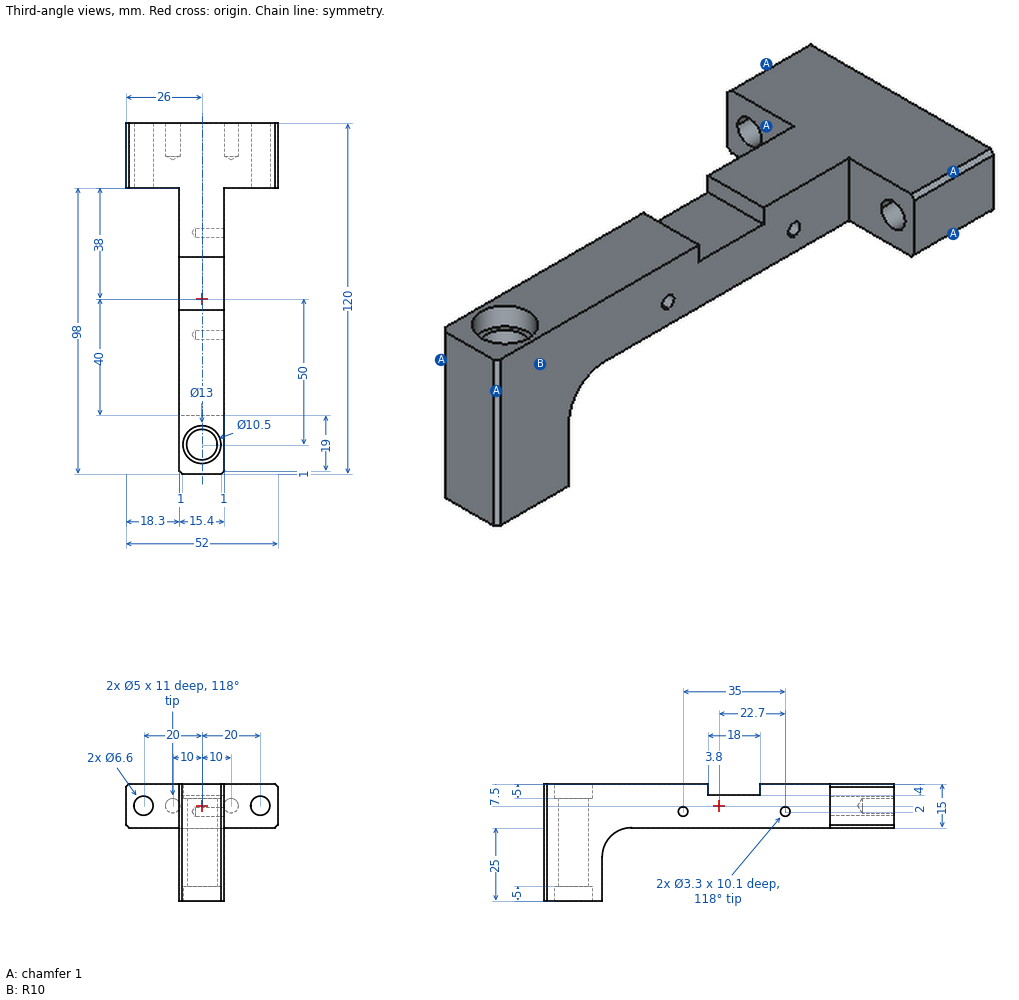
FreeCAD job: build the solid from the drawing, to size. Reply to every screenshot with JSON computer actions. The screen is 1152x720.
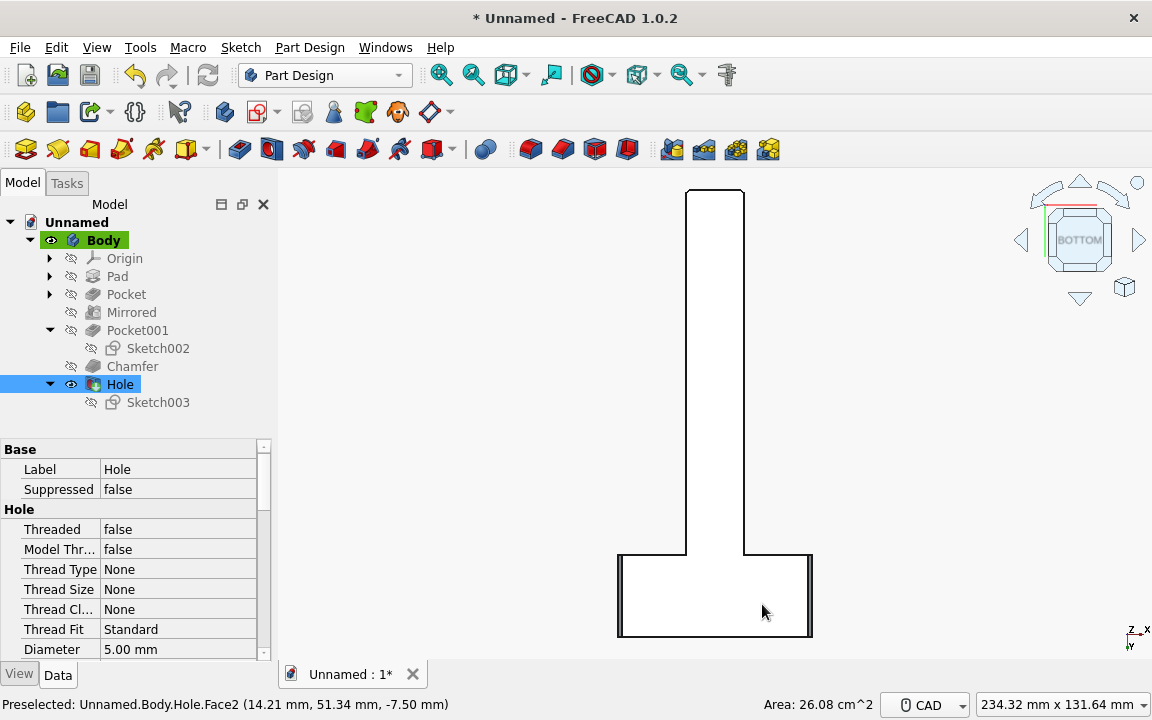
{"action": "left_click", "coordinate": [258, 112]}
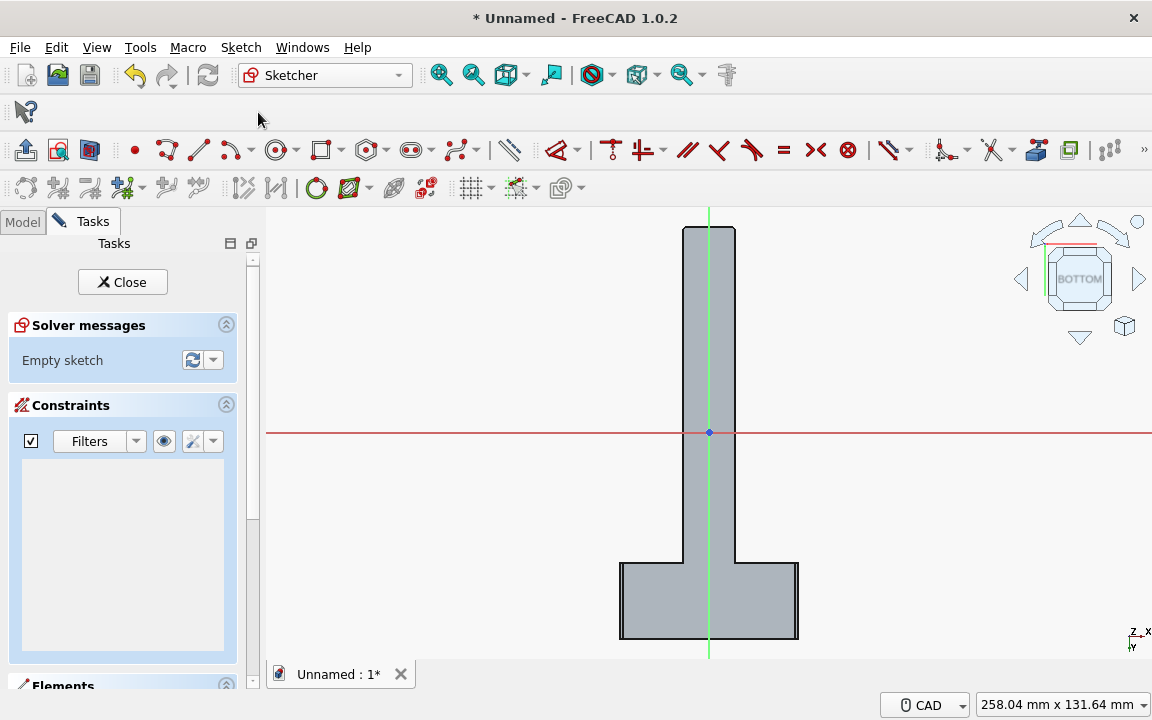
{"action": "scroll", "coordinate": [640, 433], "scroll_direction": "down", "scroll_amount": 5}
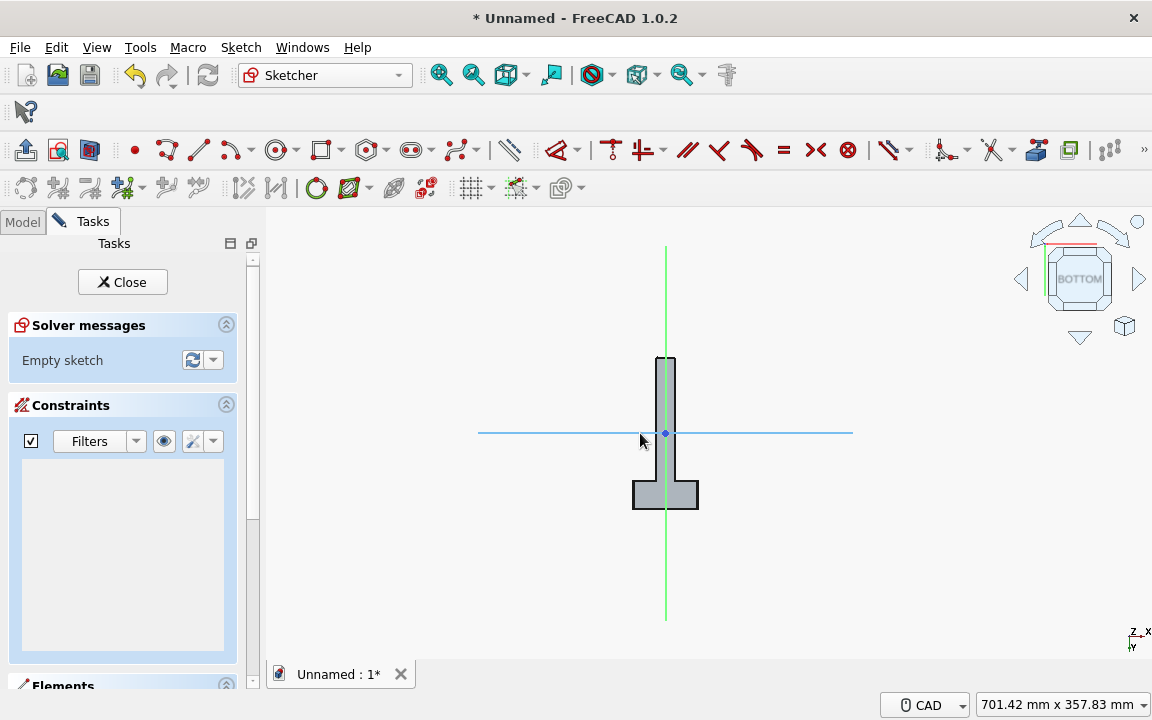
{"action": "scroll", "coordinate": [668, 364], "scroll_direction": "up", "scroll_amount": 12}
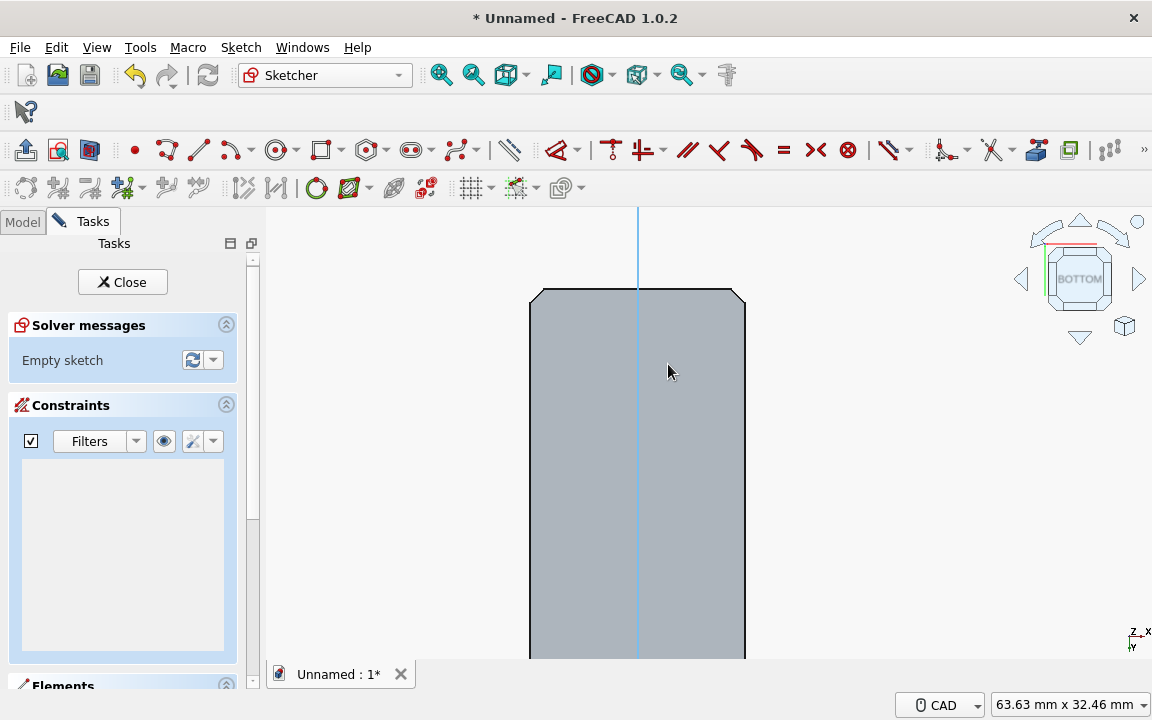
{"action": "left_click", "coordinate": [168, 150]}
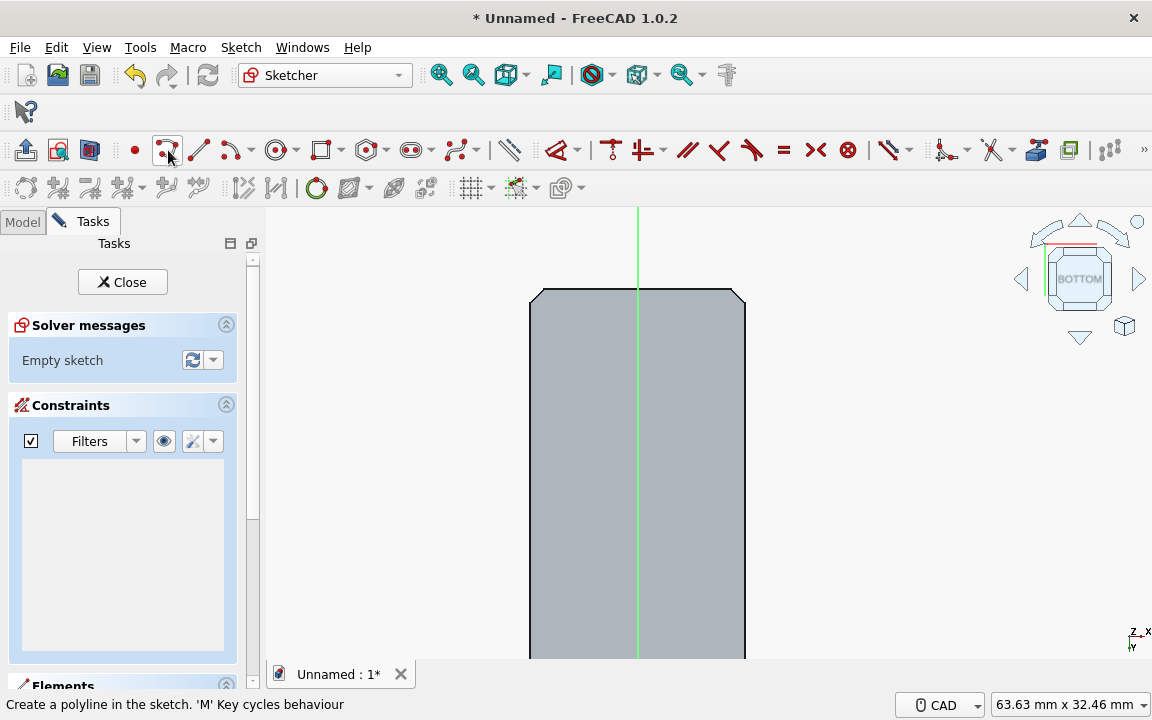
{"action": "left_click", "coordinate": [530, 568]}
{"action": "left_click", "coordinate": [745, 568]}
{"action": "left_click", "coordinate": [745, 303]}
{"action": "left_click", "coordinate": [731, 289]}
{"action": "left_click", "coordinate": [544, 289]}
{"action": "left_click", "coordinate": [530, 303]}
{"action": "left_click", "coordinate": [530, 569]}
{"action": "key", "text": "Escape"}
{"action": "key", "text": "Escape"}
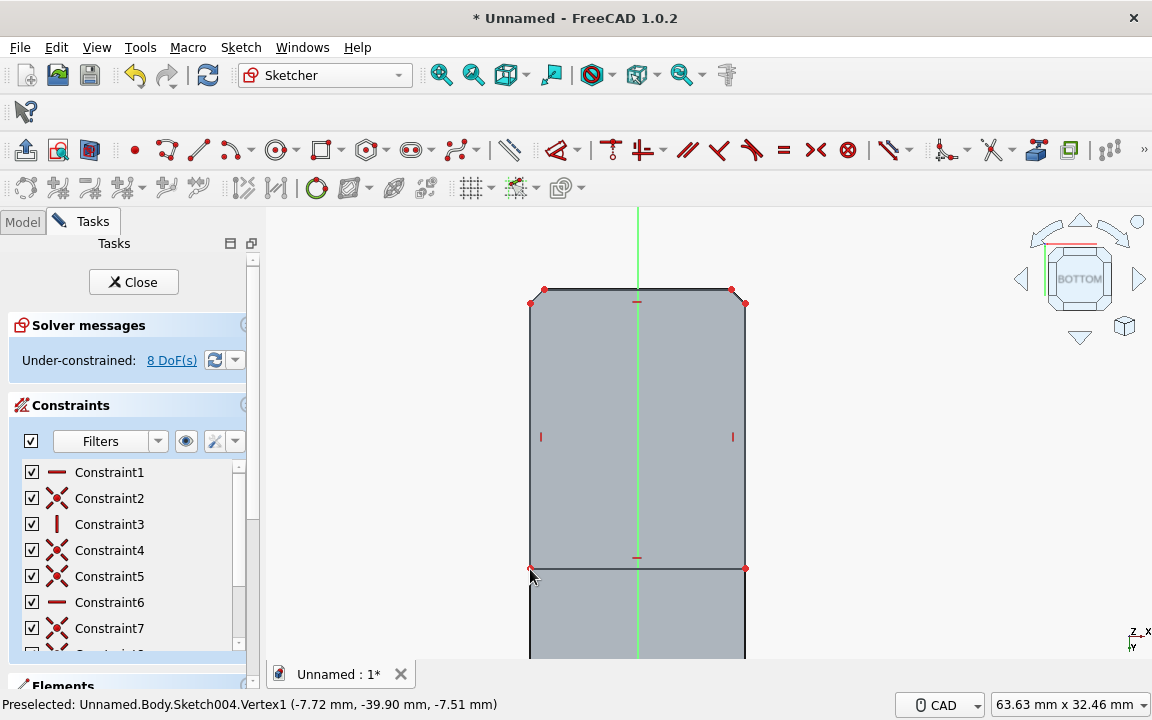
{"action": "left_click", "coordinate": [745, 304]}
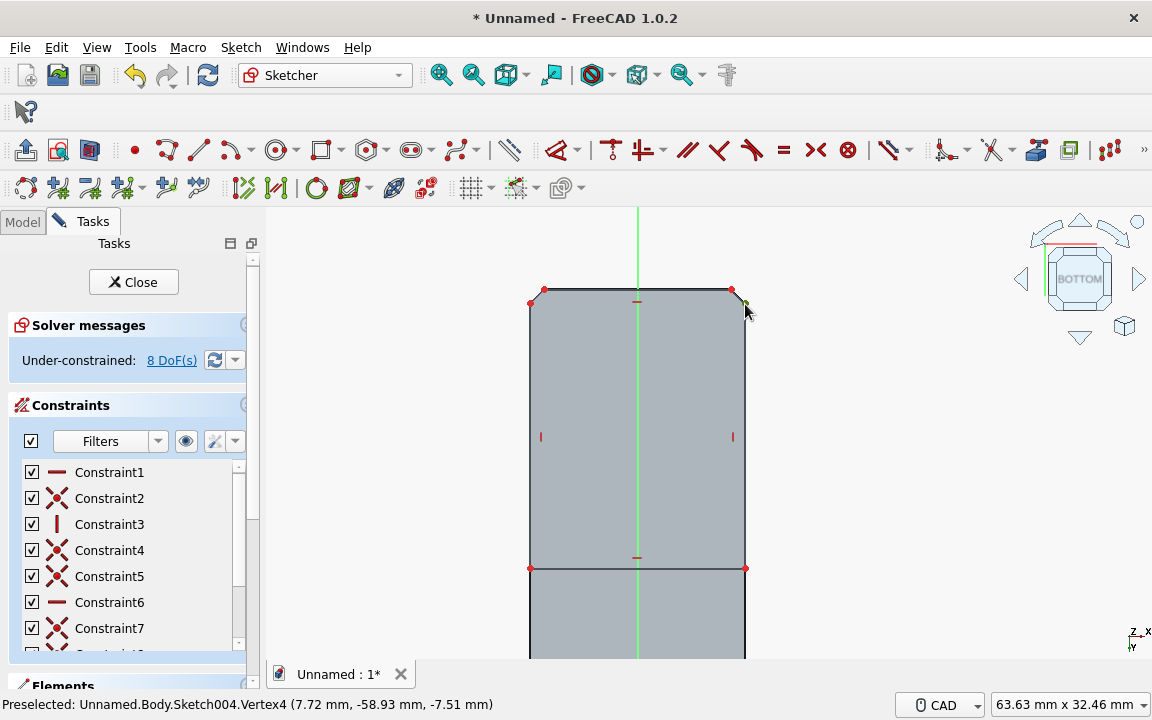
{"action": "left_click", "coordinate": [530, 304]}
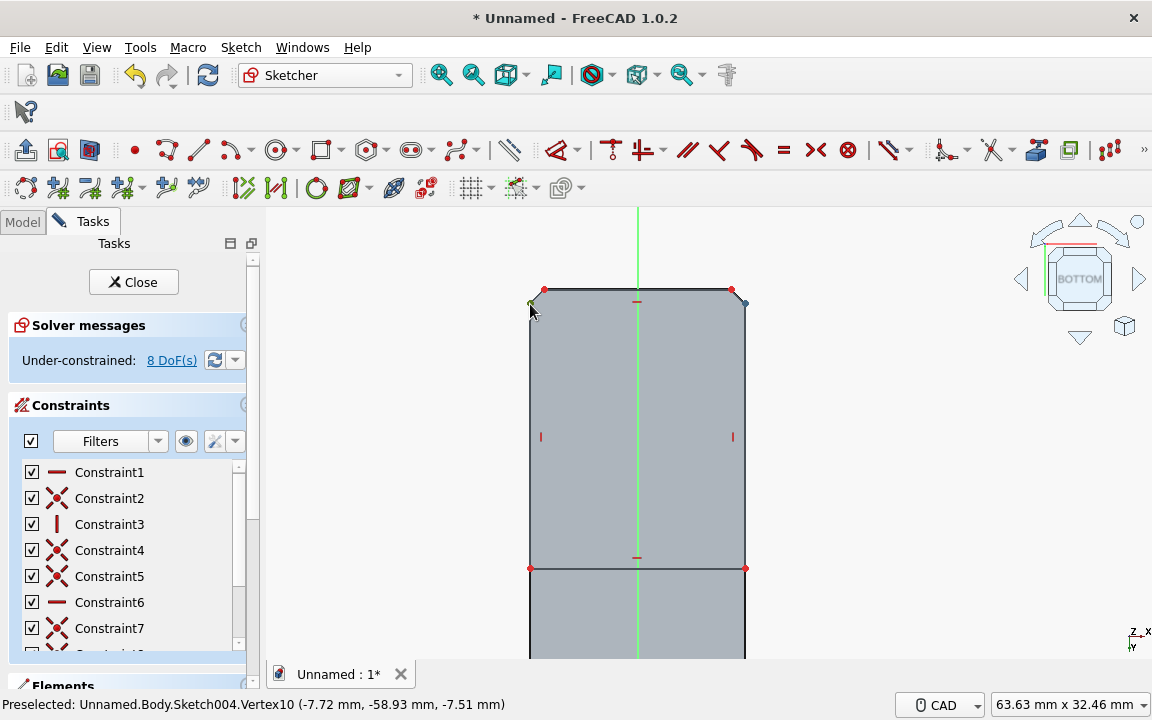
{"action": "left_click", "coordinate": [638, 603]}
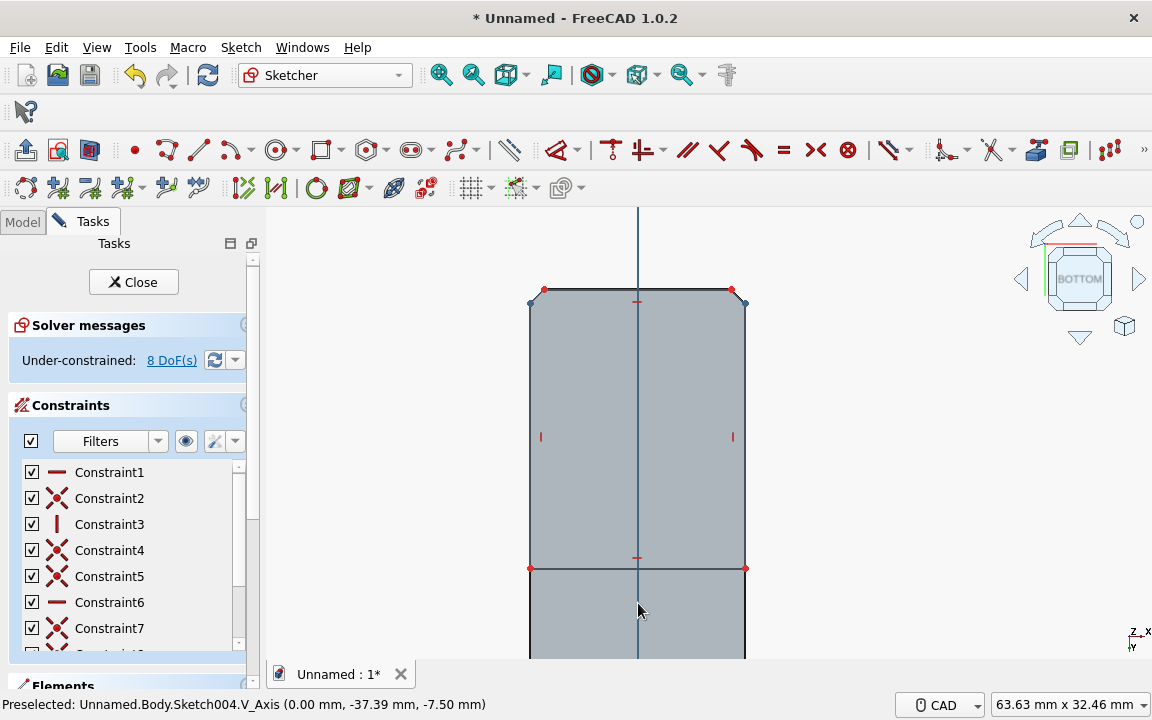
{"action": "left_click", "coordinate": [816, 150]}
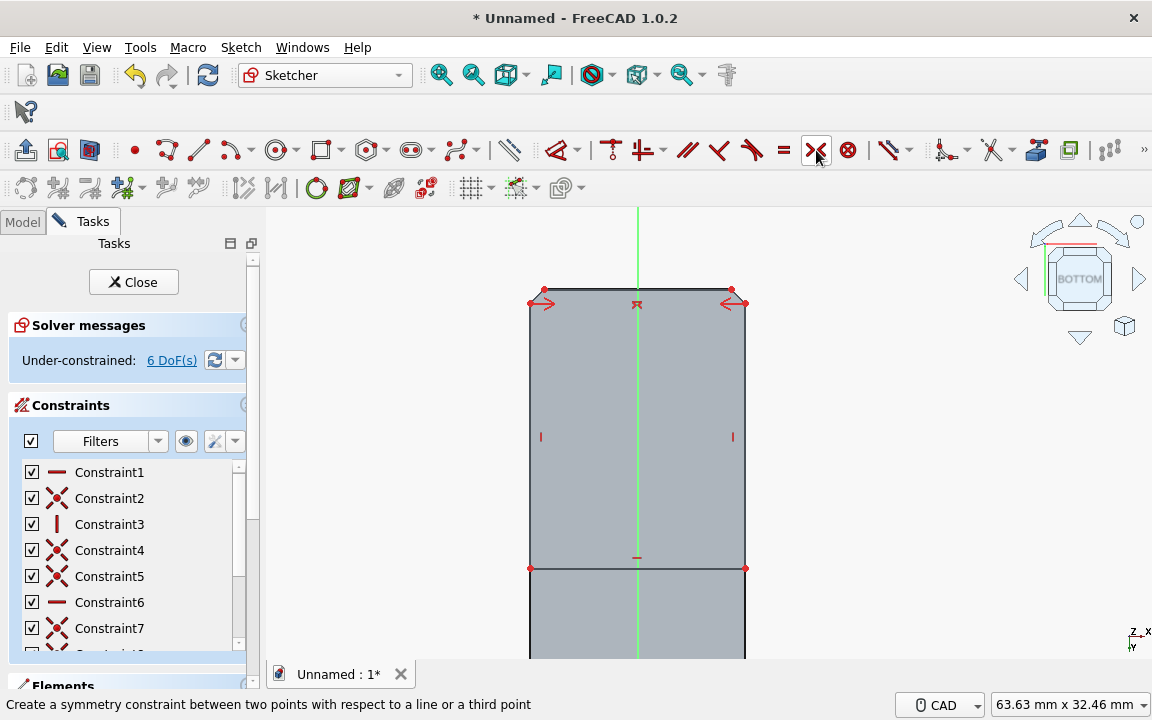
{"action": "left_click", "coordinate": [556, 150]}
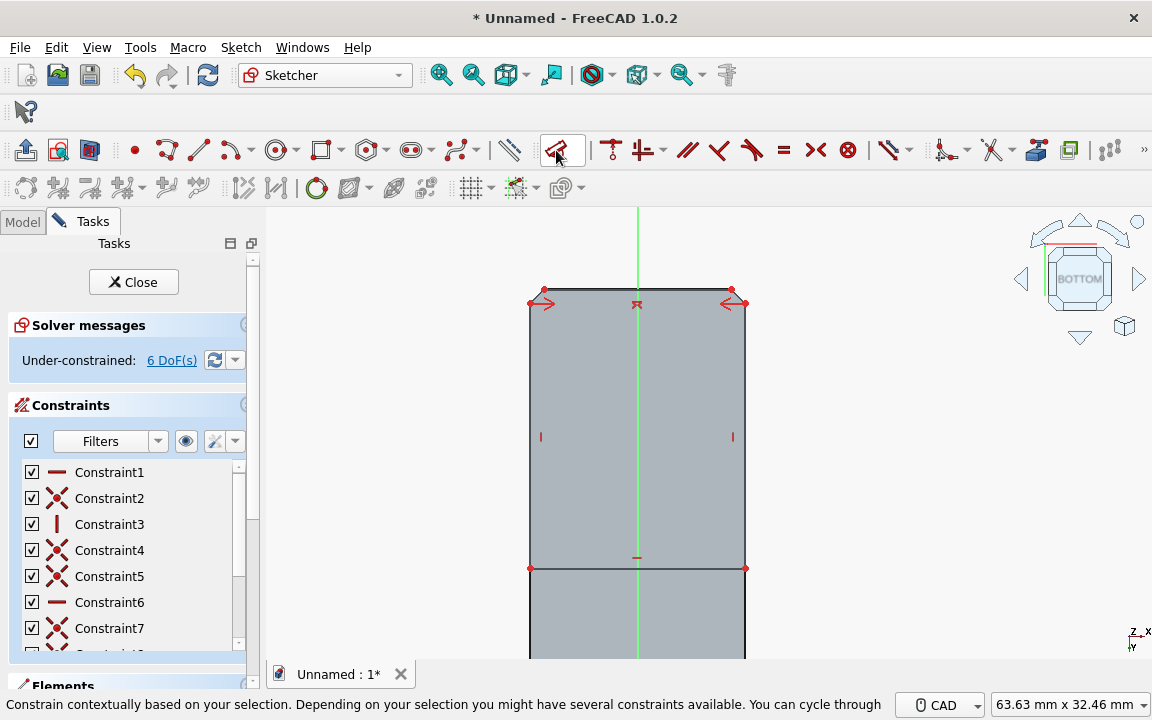
{"action": "left_click", "coordinate": [745, 490]}
{"action": "left_click", "coordinate": [779, 437]}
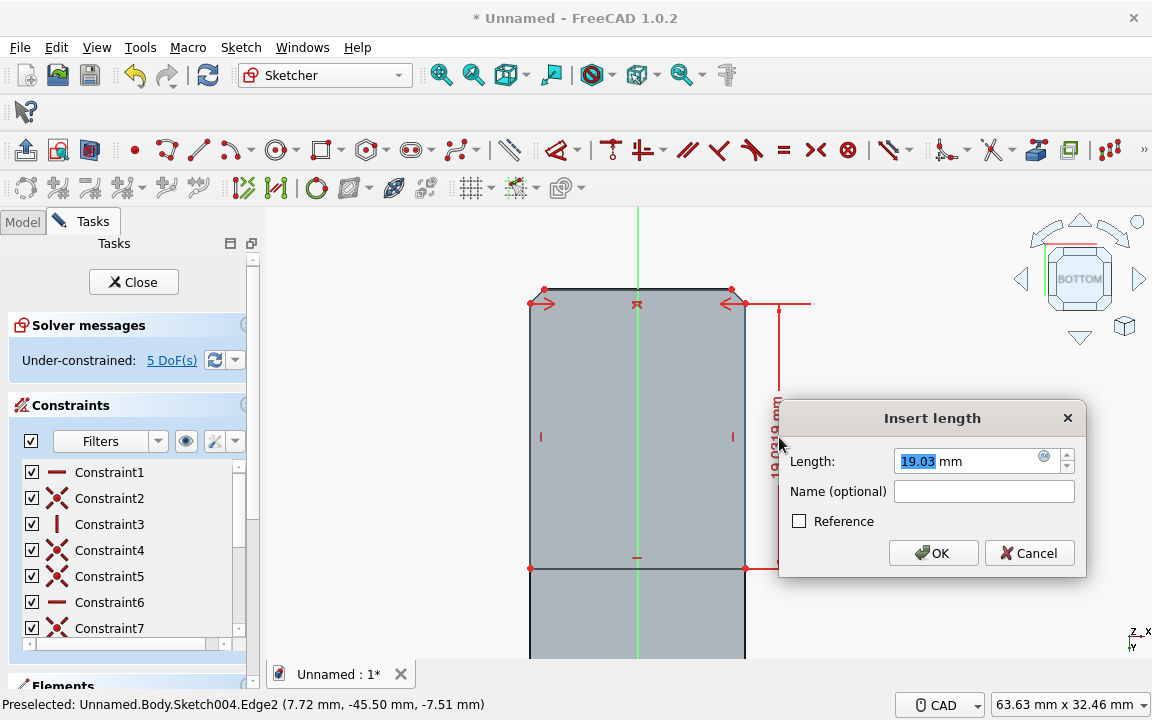
{"action": "type", "text": "19"}
{"action": "key", "text": "Return"}